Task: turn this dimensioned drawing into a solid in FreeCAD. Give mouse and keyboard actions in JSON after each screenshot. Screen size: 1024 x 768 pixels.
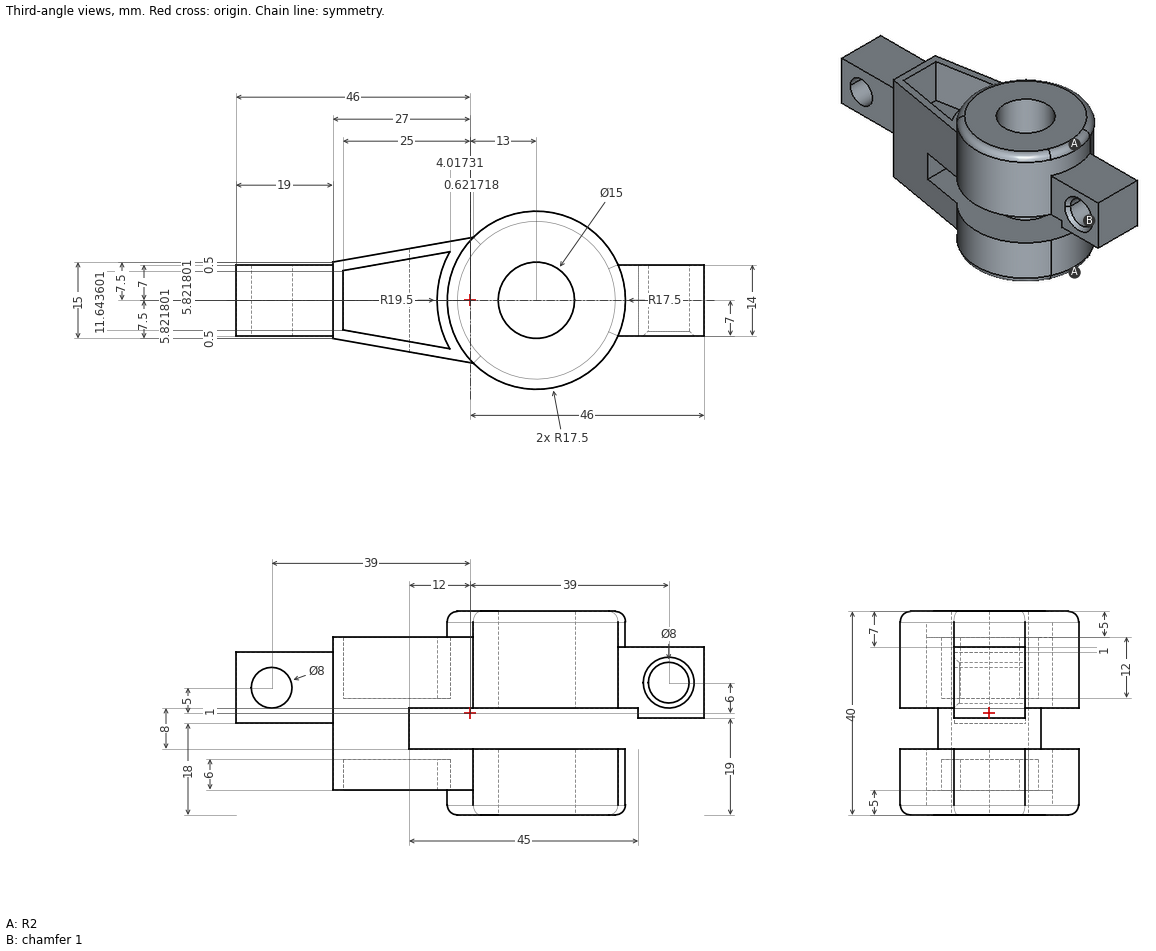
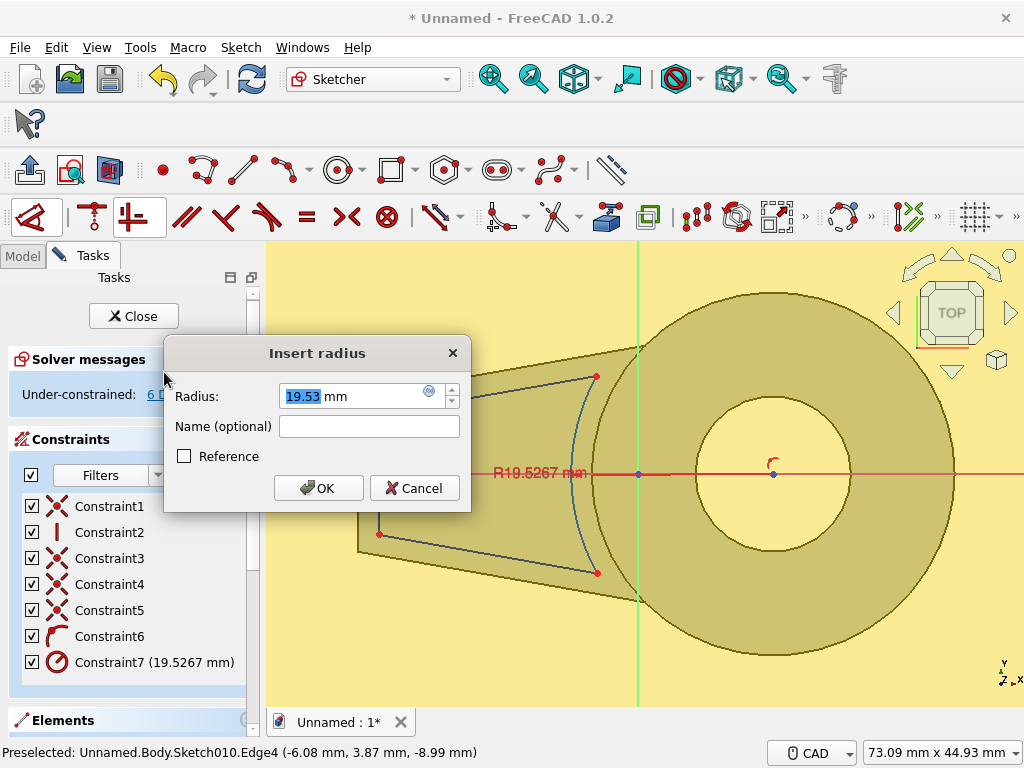
{"action": "type", "text": "19.5"}
{"action": "key", "text": "Return"}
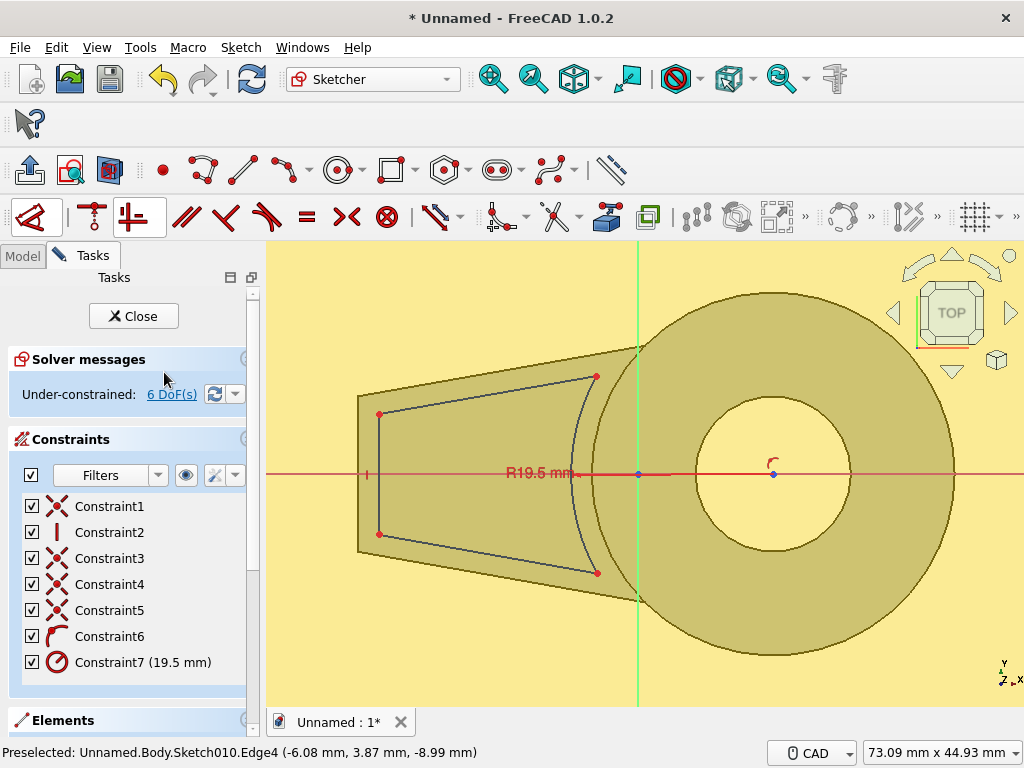
{"action": "left_click", "coordinate": [379, 535]}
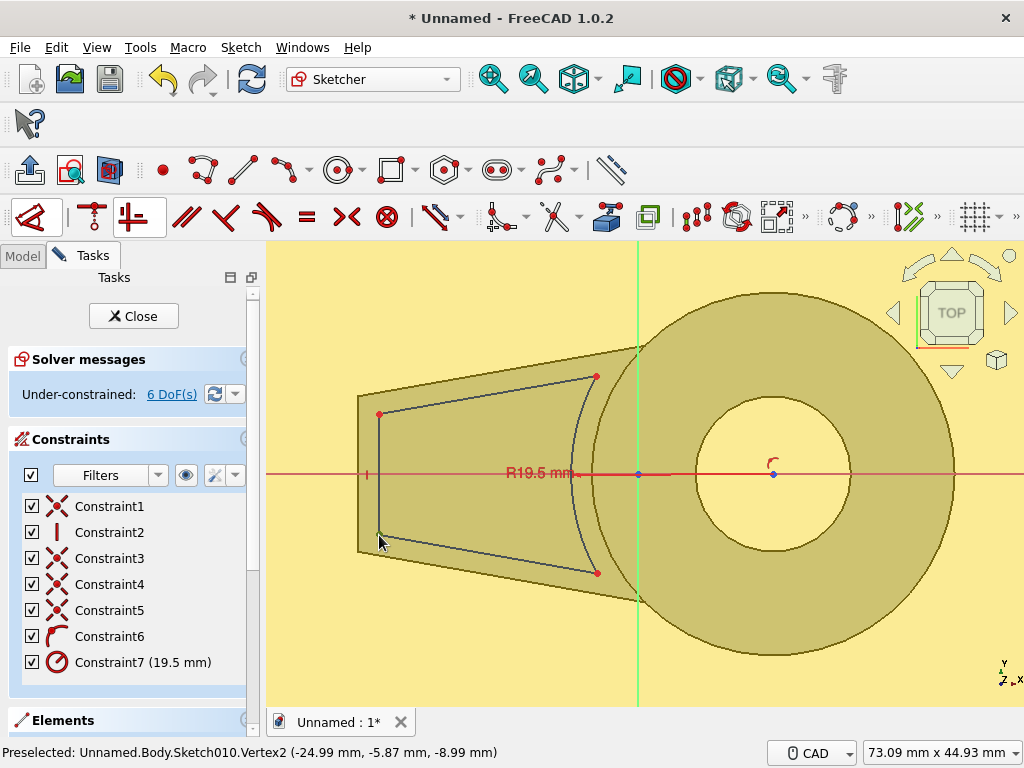
{"action": "key", "text": "l"}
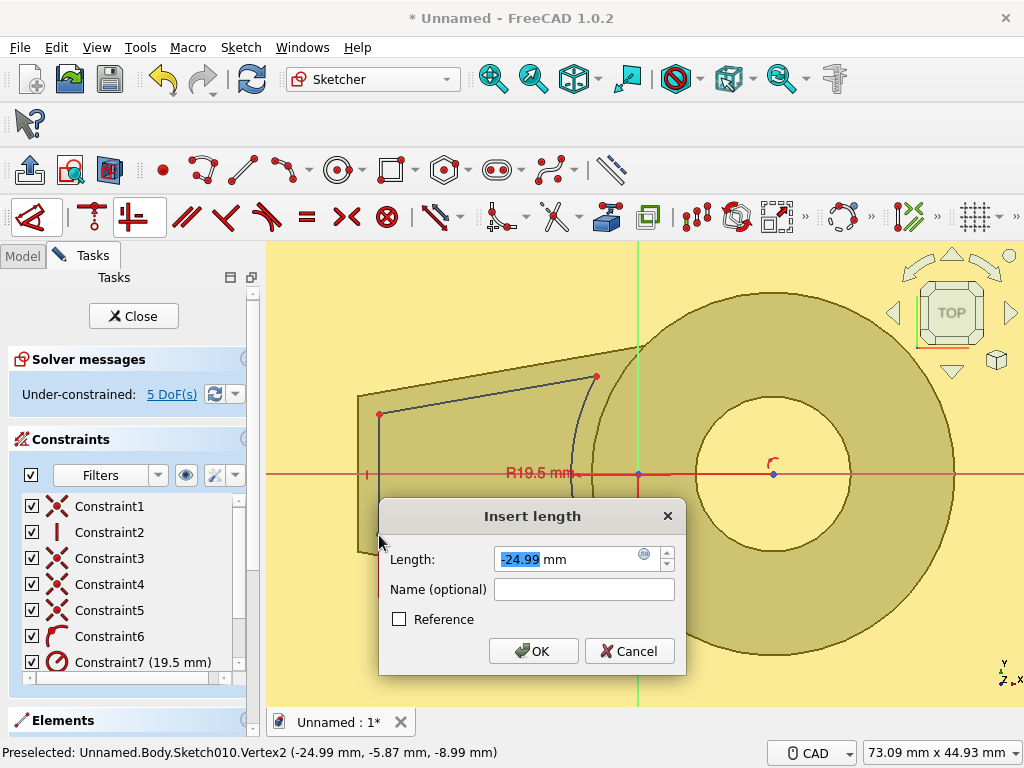
{"action": "type", "text": "-25"}
{"action": "key", "text": "Return"}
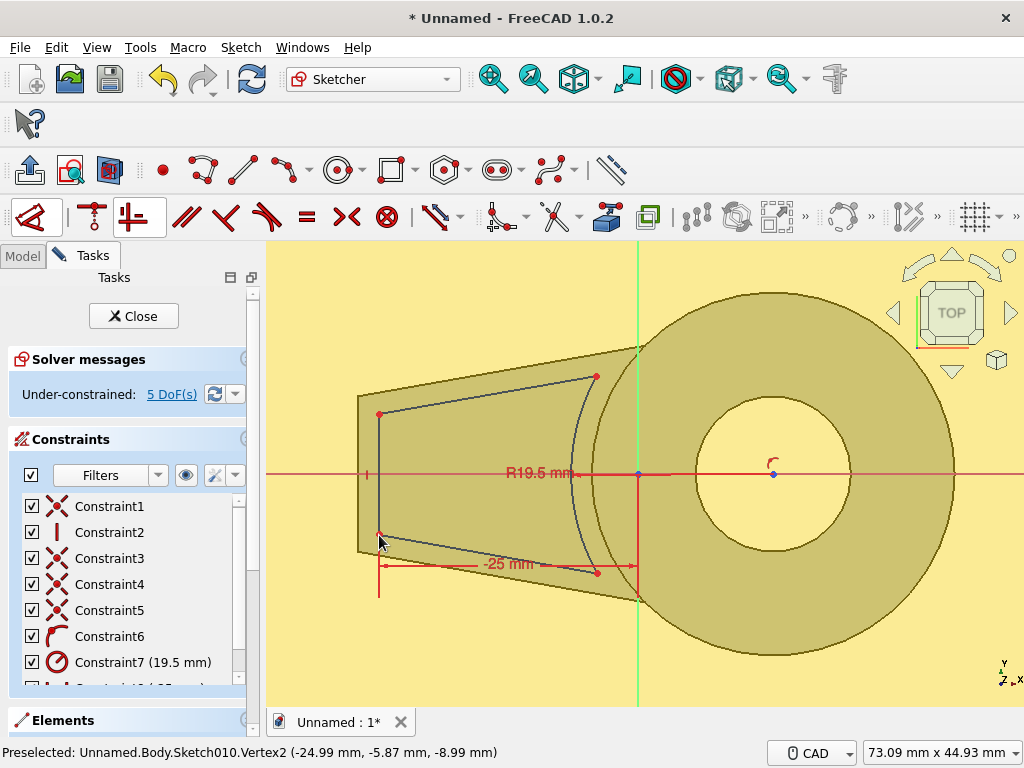
{"action": "left_click", "coordinate": [773, 474]}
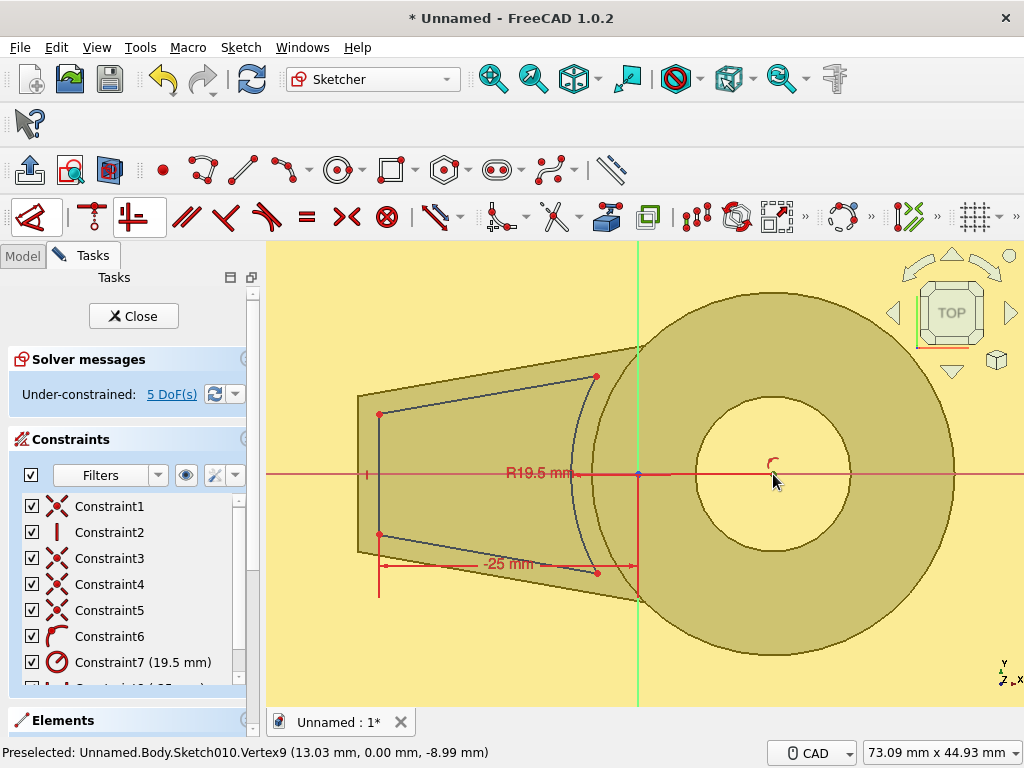
{"action": "left_click", "coordinate": [56, 218]}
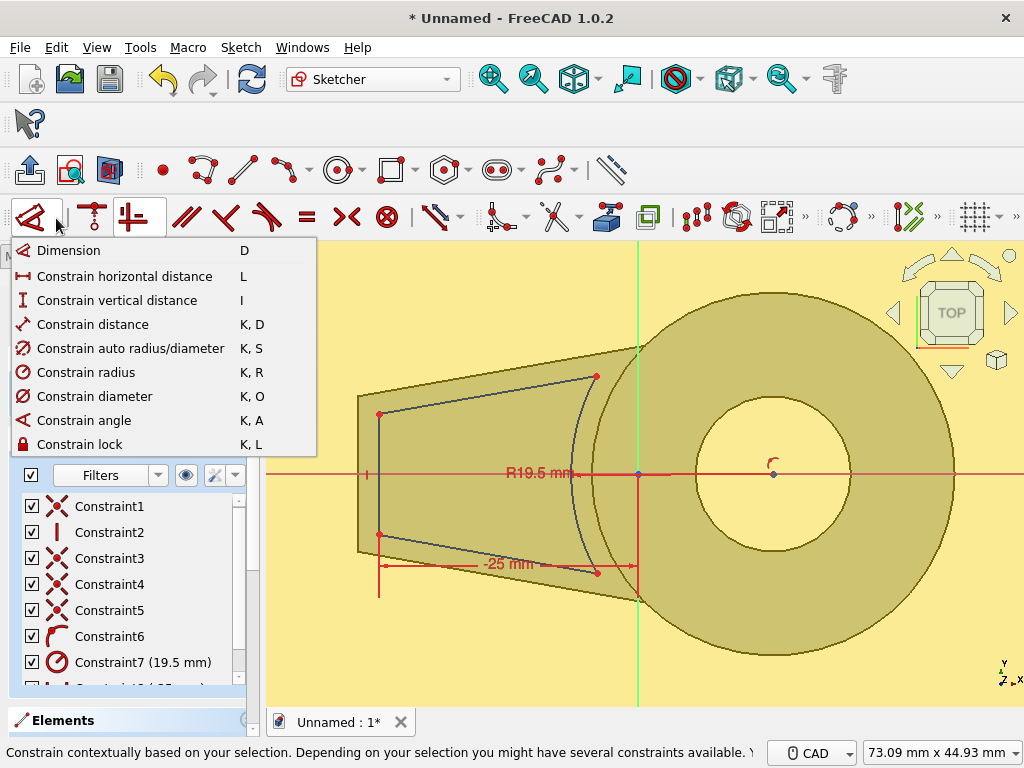
{"action": "left_click", "coordinate": [164, 276]}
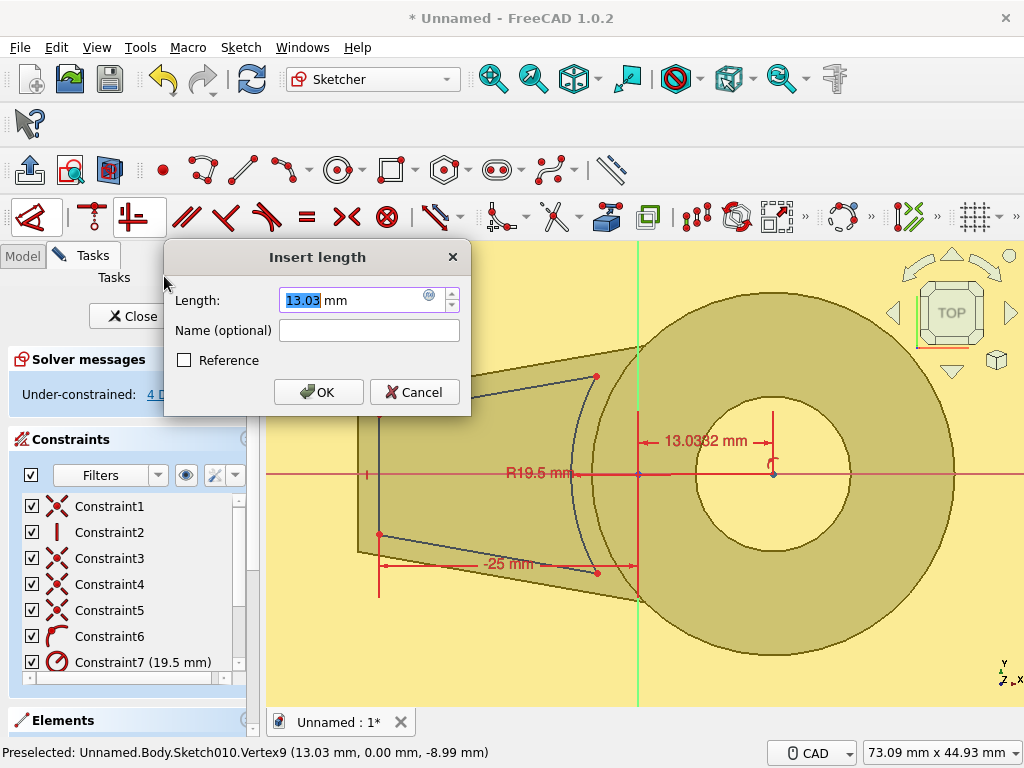
{"action": "type", "text": "13"}
{"action": "key", "text": "Return"}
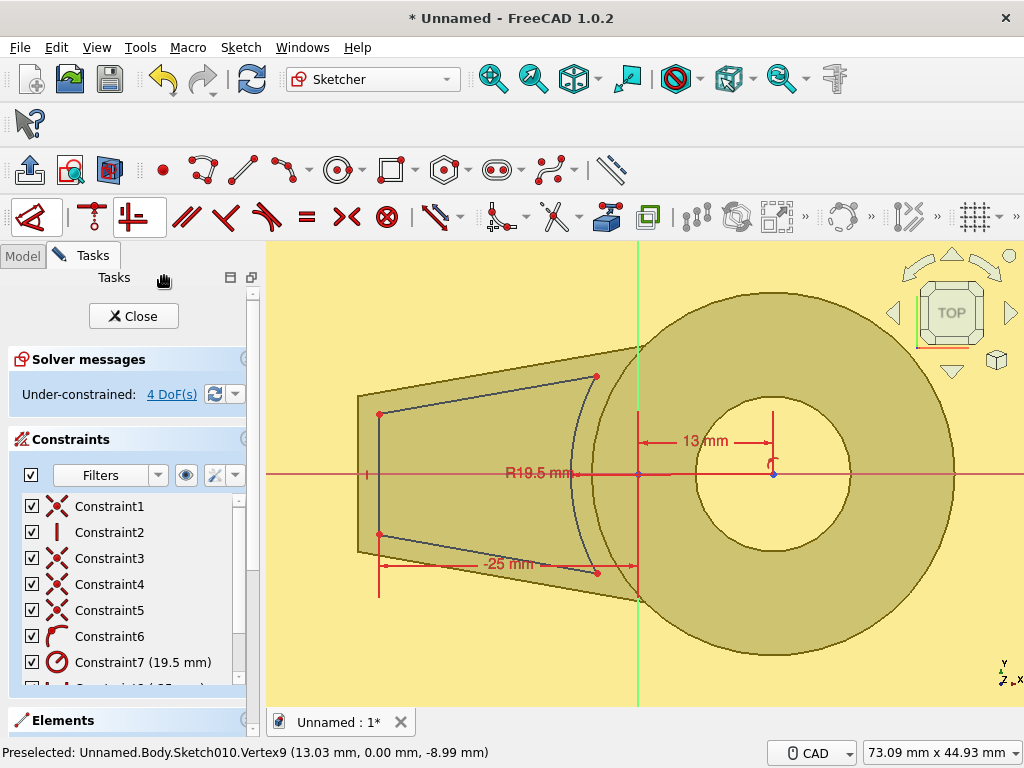
{"action": "left_click", "coordinate": [597, 574]}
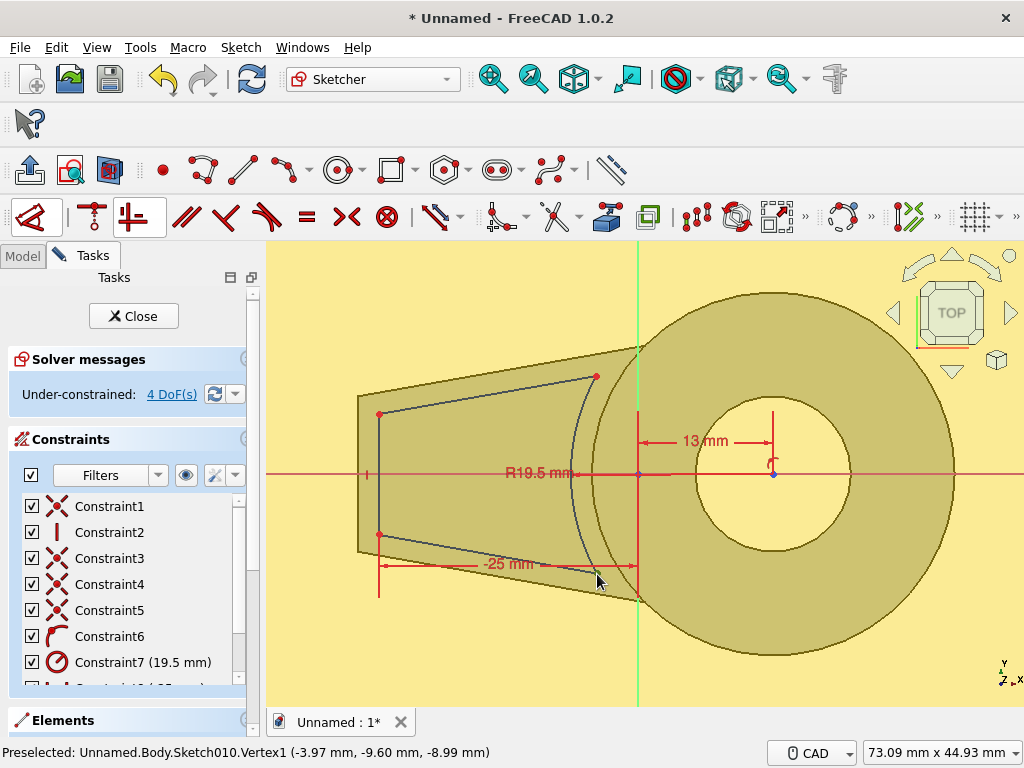
{"action": "left_click", "coordinate": [56, 218]}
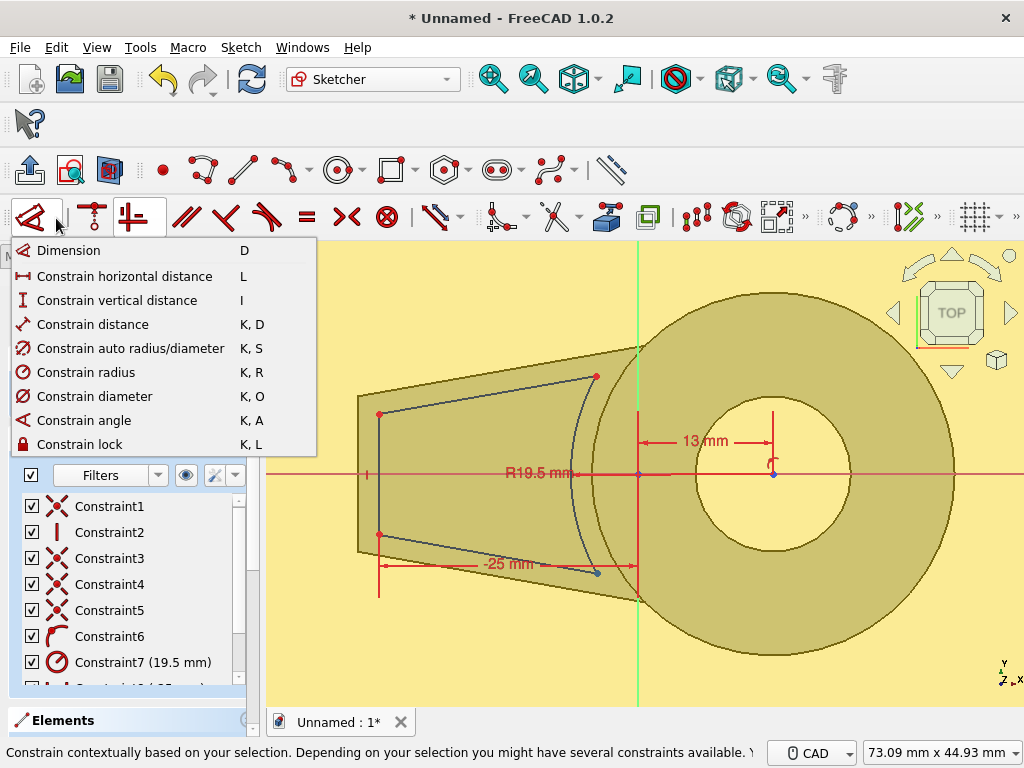
{"action": "left_click", "coordinate": [164, 276]}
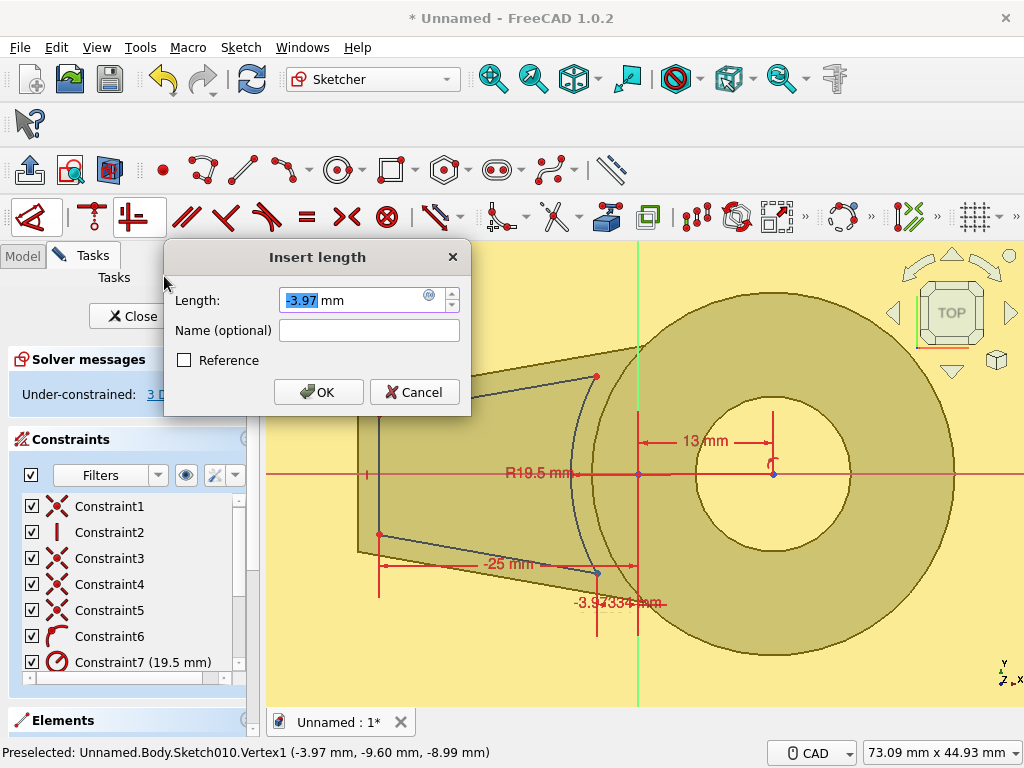
{"action": "type", "text": "-4.01731"}
{"action": "key", "text": "Return"}